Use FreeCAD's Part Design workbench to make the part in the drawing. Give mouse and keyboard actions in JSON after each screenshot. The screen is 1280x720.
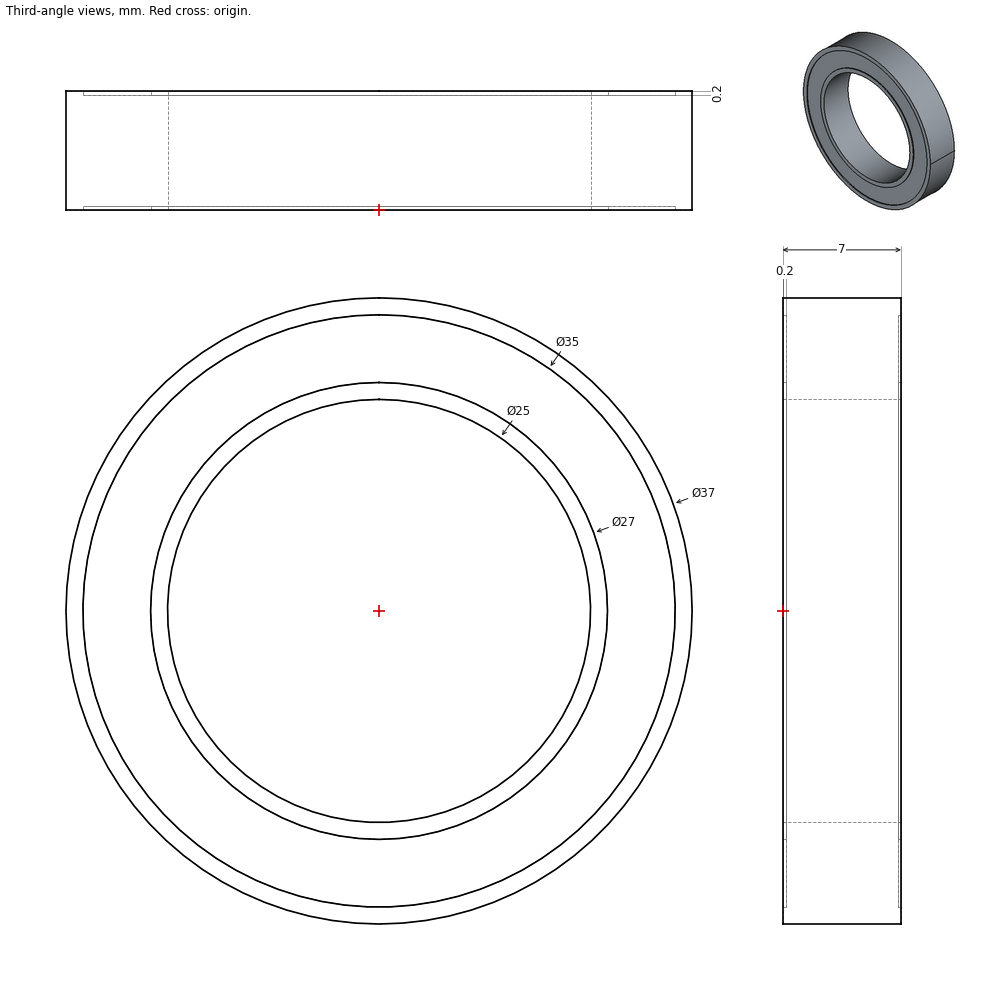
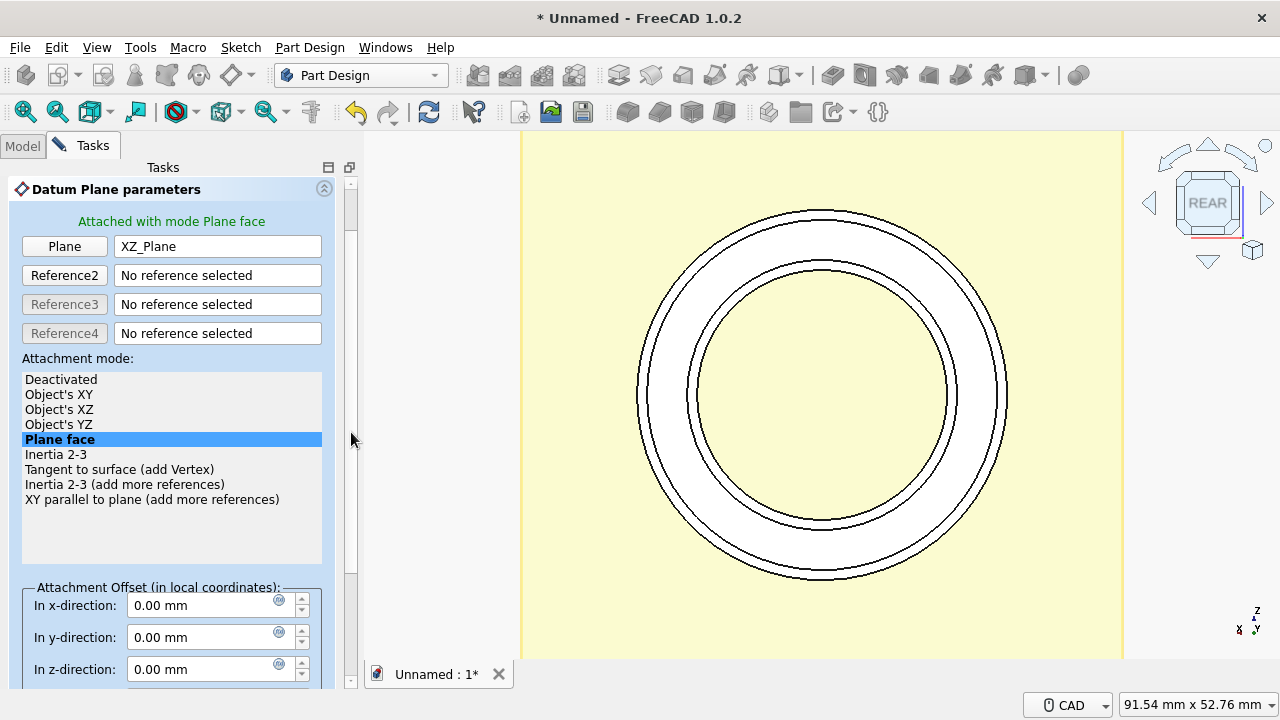
{"action": "triple_click", "coordinate": [210, 609]}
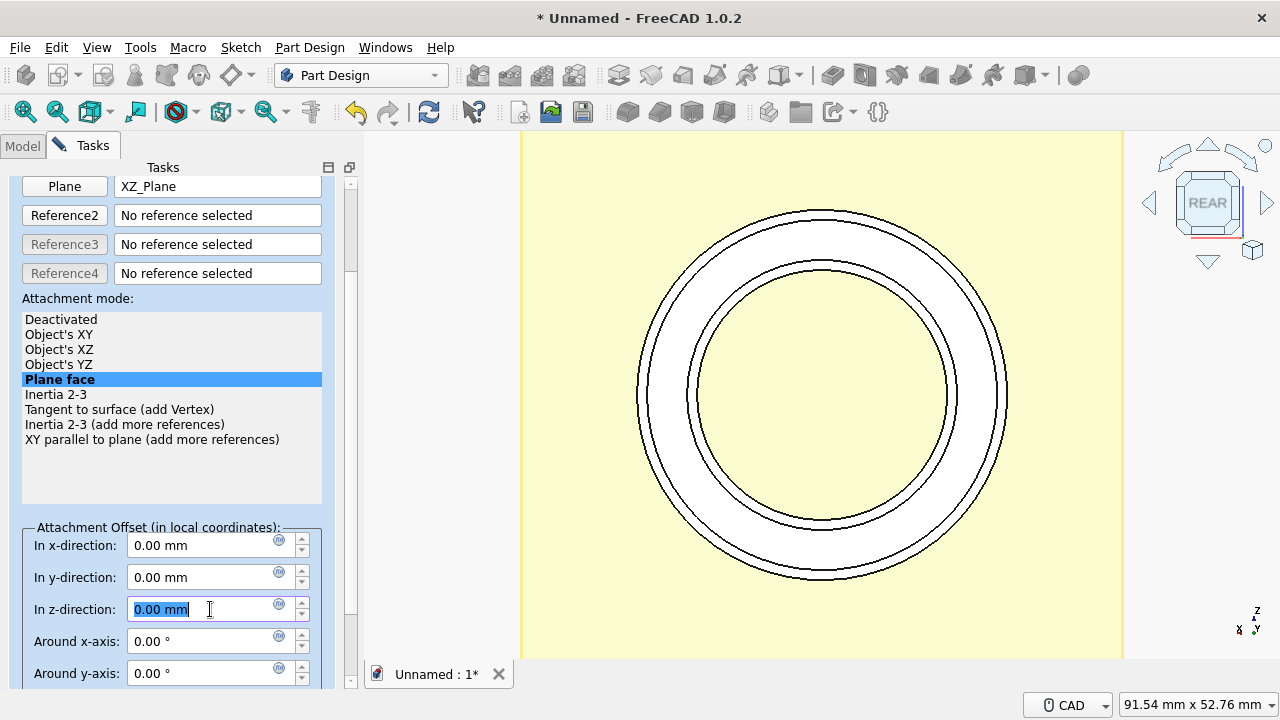
{"action": "type", "text": "-0.2"}
{"action": "key", "text": "Tab"}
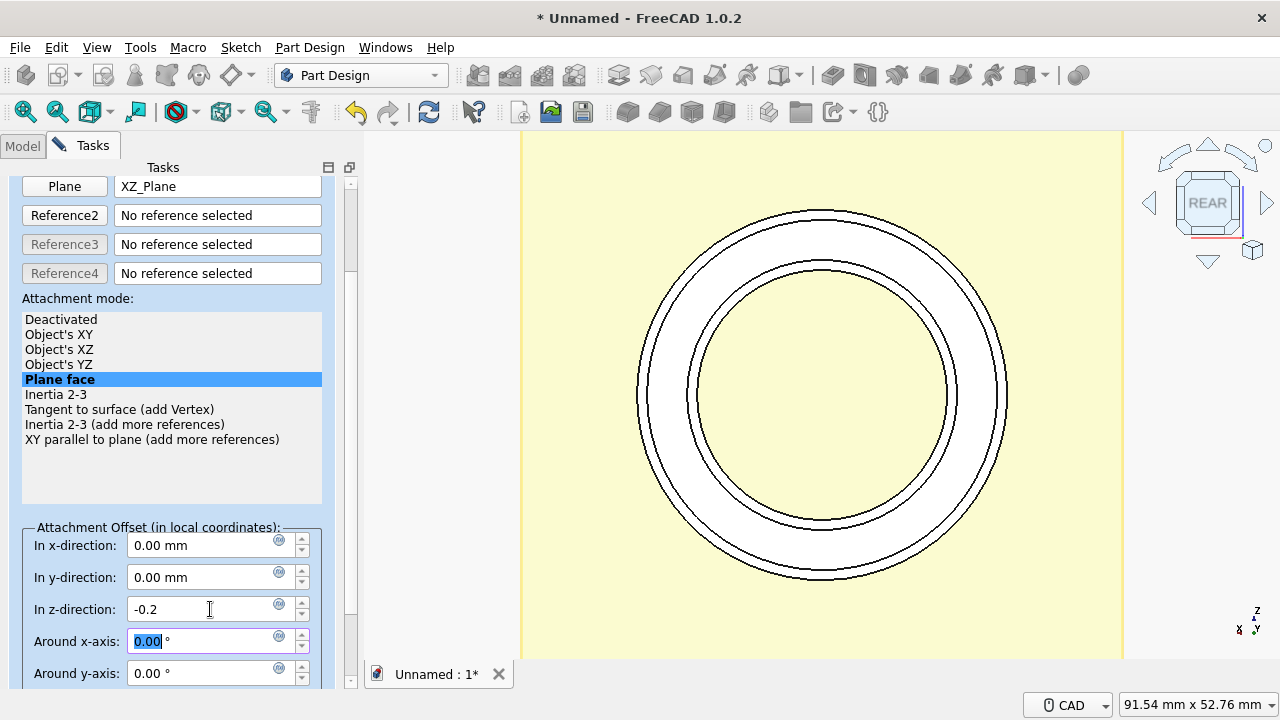
{"action": "scroll", "coordinate": [351, 432], "scroll_direction": "up", "scroll_amount": 3}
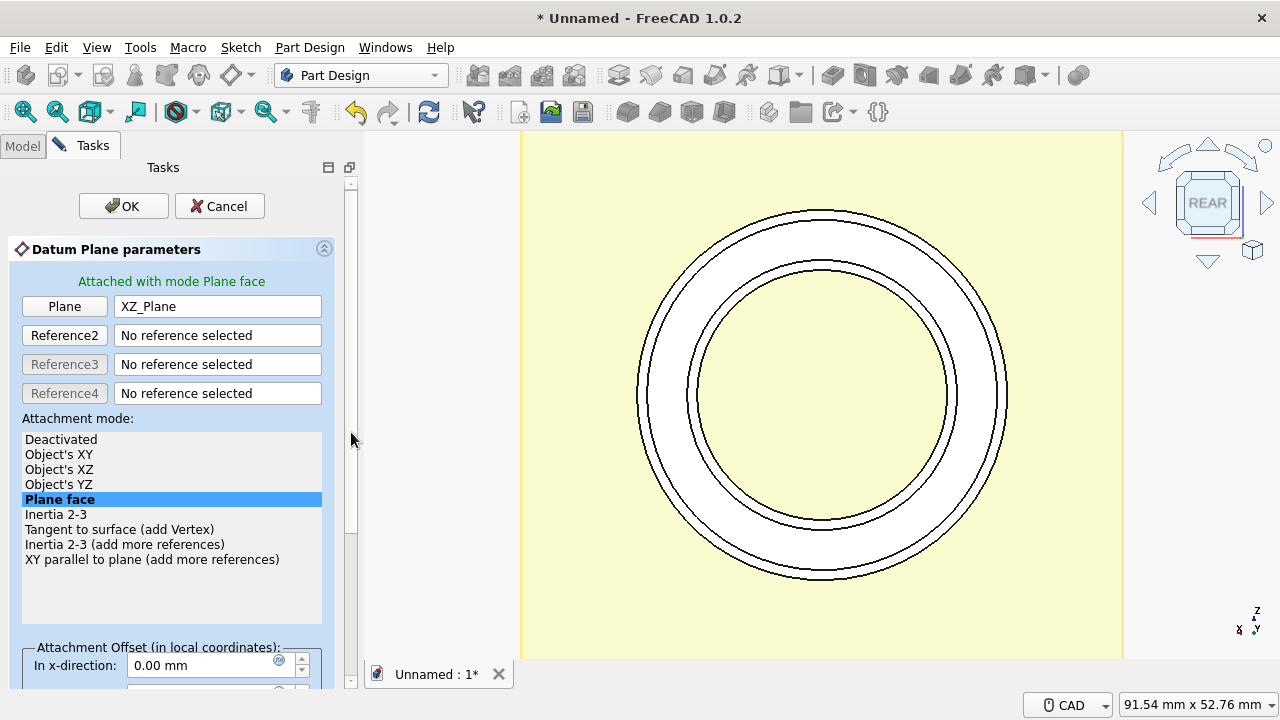
{"action": "left_click", "coordinate": [124, 206]}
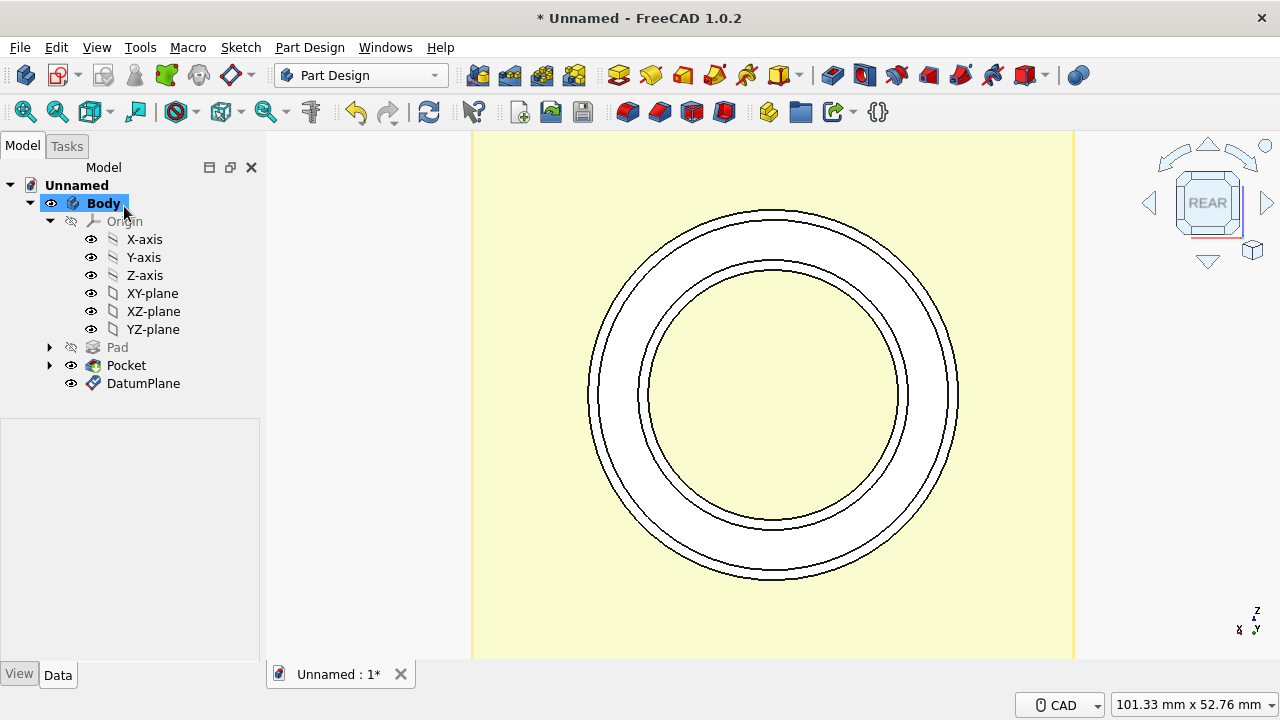
{"action": "left_click", "coordinate": [116, 383]}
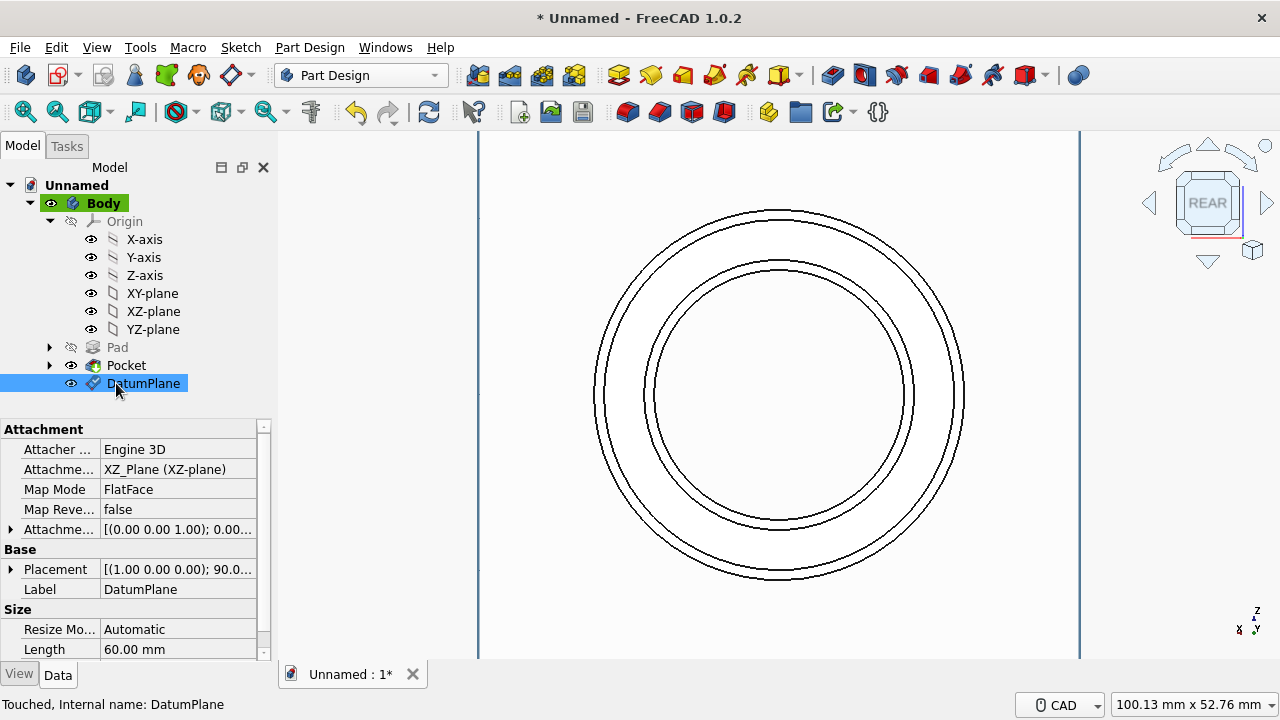
{"action": "left_click", "coordinate": [58, 76]}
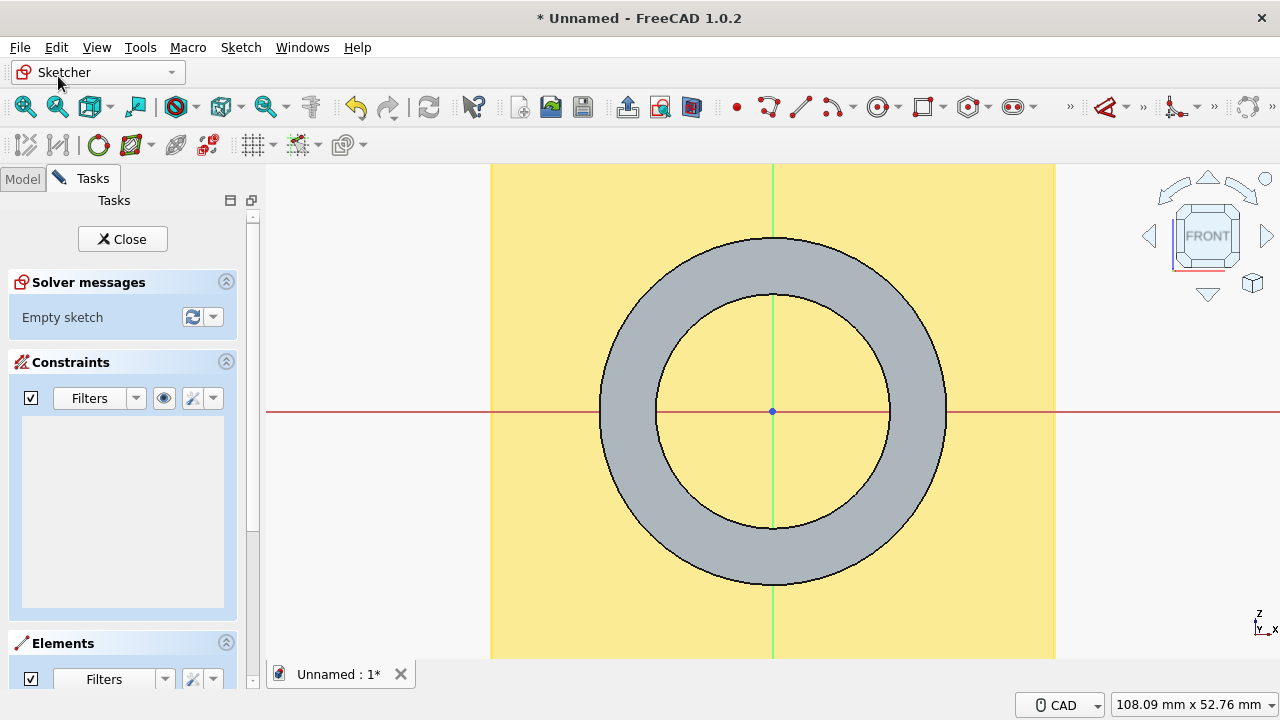
{"action": "left_click", "coordinate": [692, 108]}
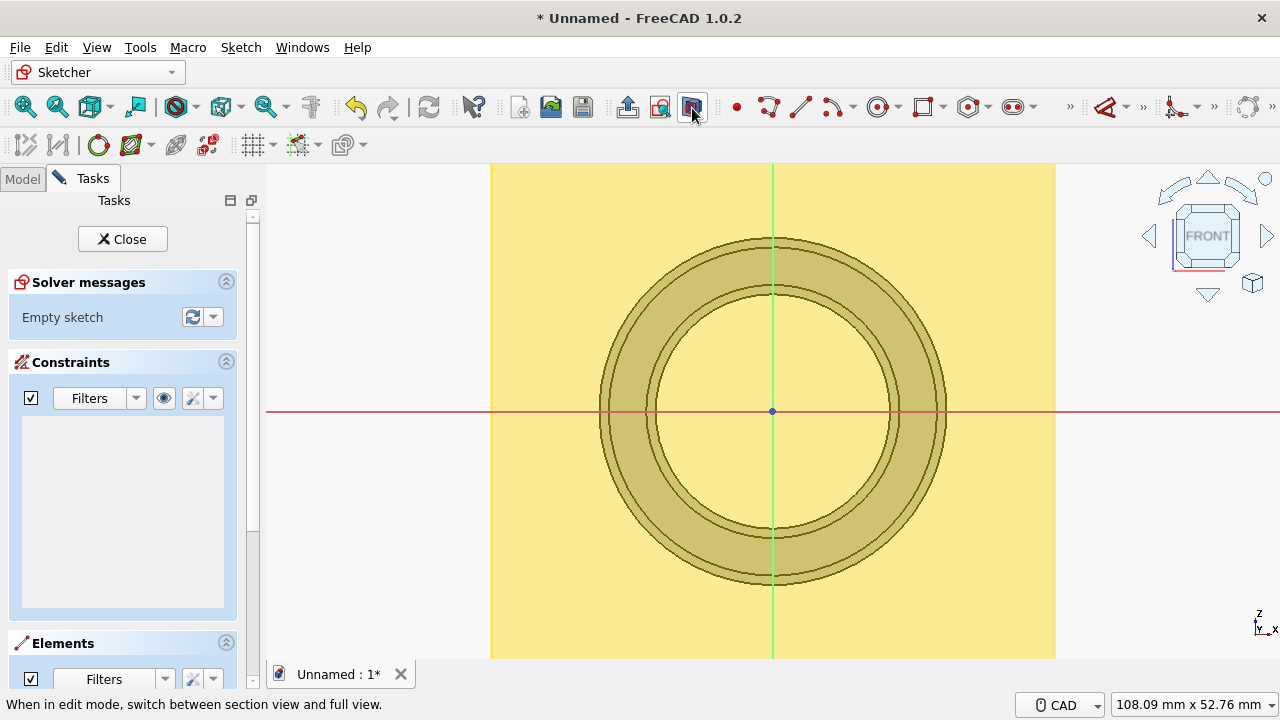
{"action": "key", "text": "g c"}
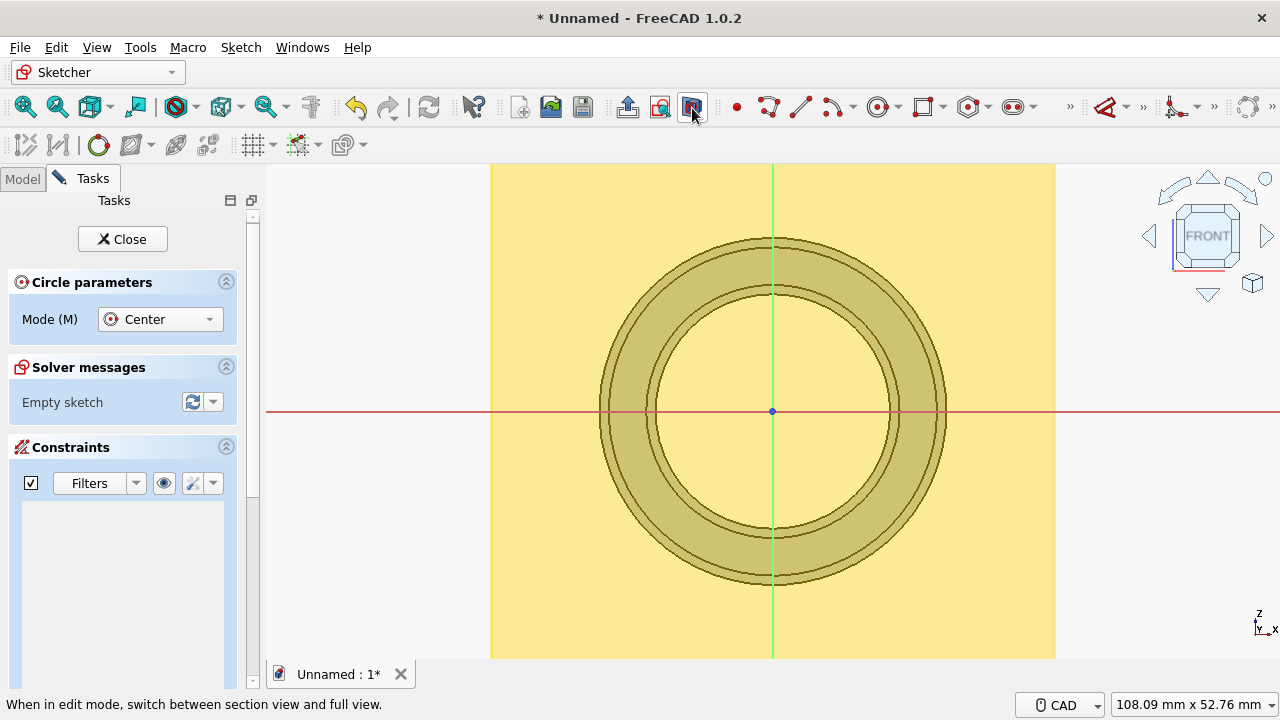
{"action": "left_click", "coordinate": [773, 412]}
{"action": "mouse_move", "coordinate": [889, 295]}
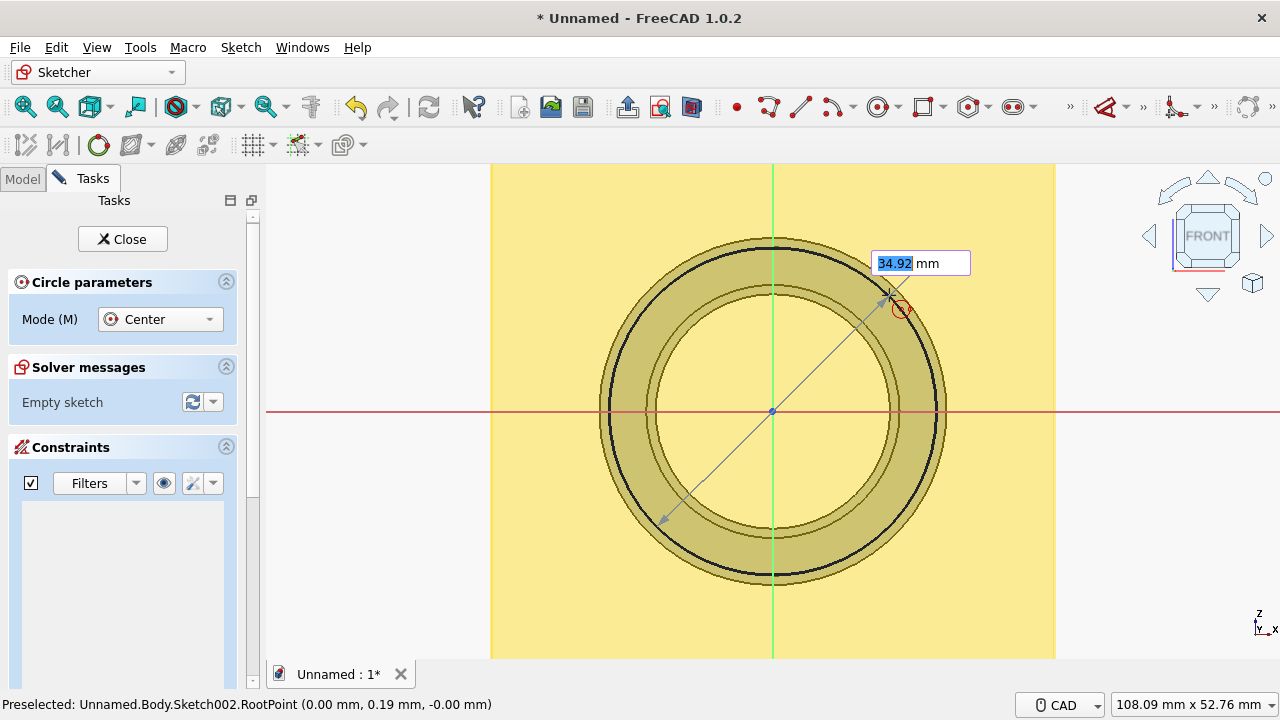
{"action": "type", "text": "35"}
{"action": "key", "text": "Return"}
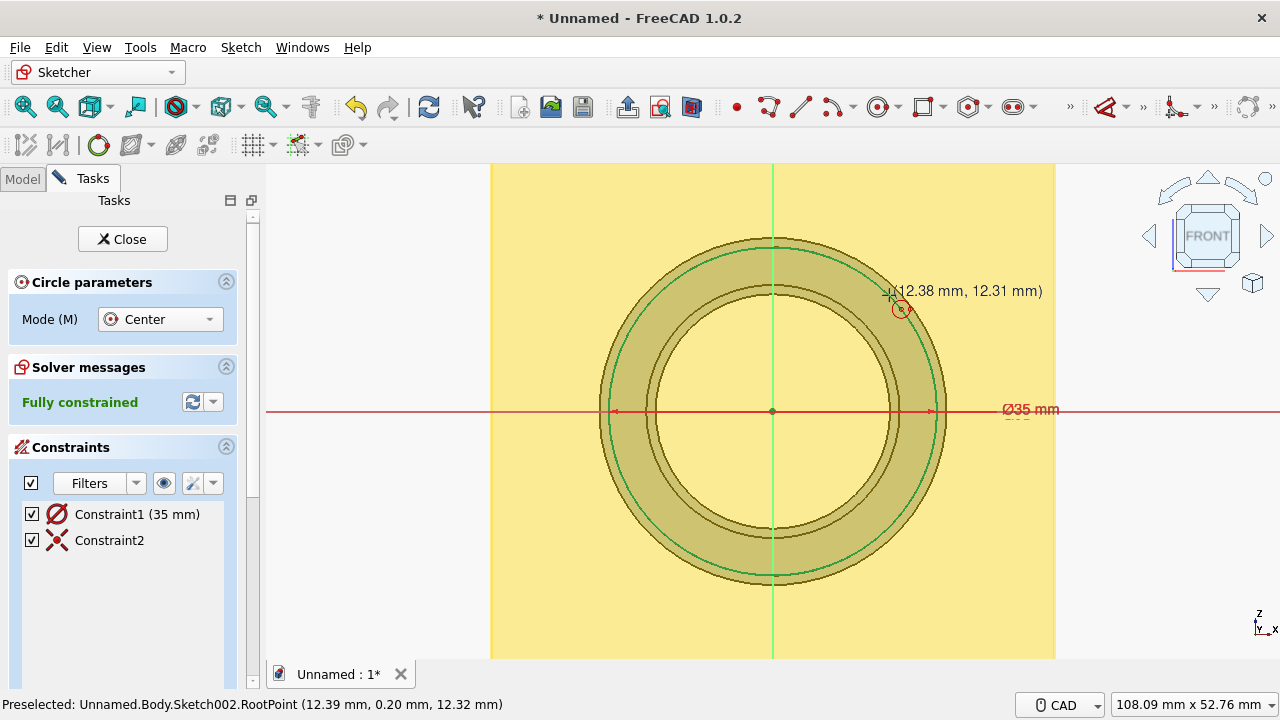
{"action": "left_click", "coordinate": [773, 412]}
{"action": "mouse_move", "coordinate": [862, 322]}